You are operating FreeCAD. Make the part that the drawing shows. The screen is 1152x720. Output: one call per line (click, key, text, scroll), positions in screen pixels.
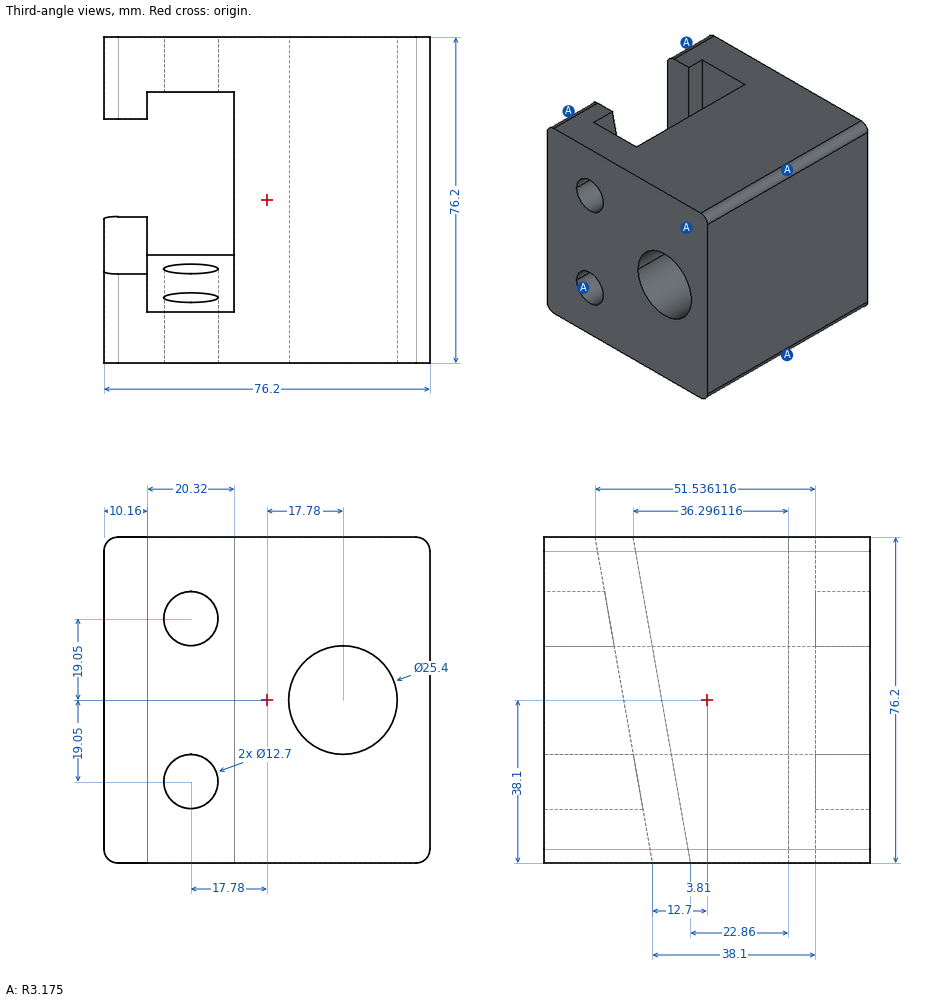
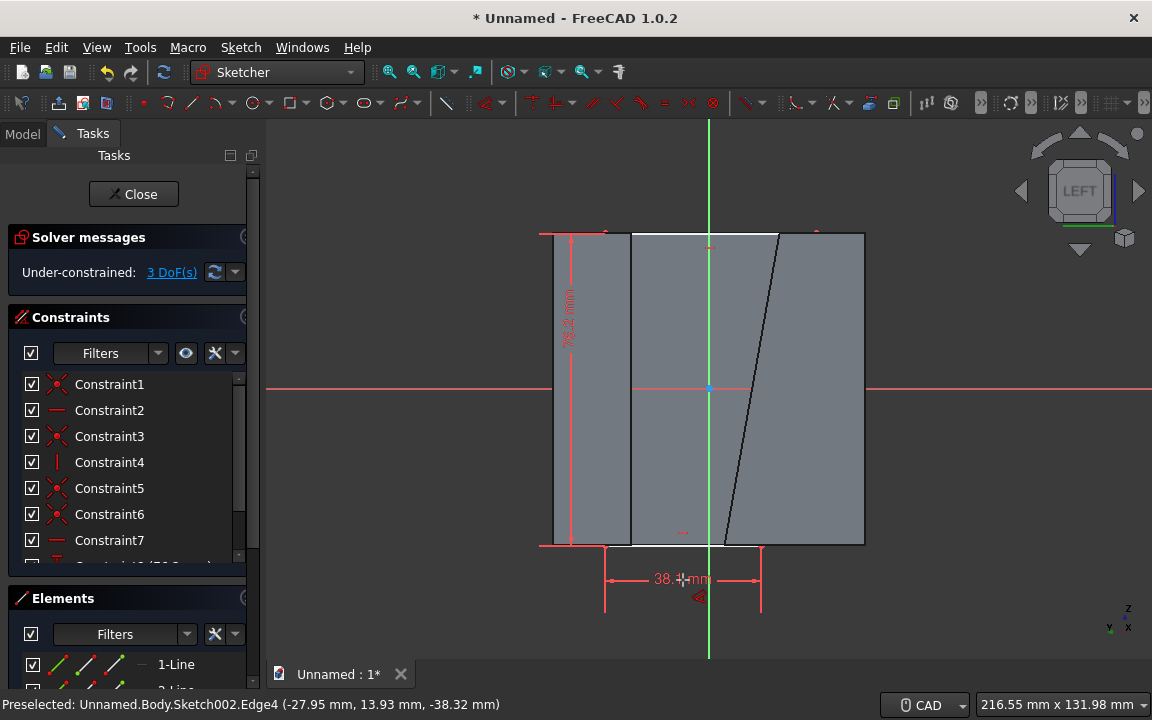
click(761, 546)
click(753, 580)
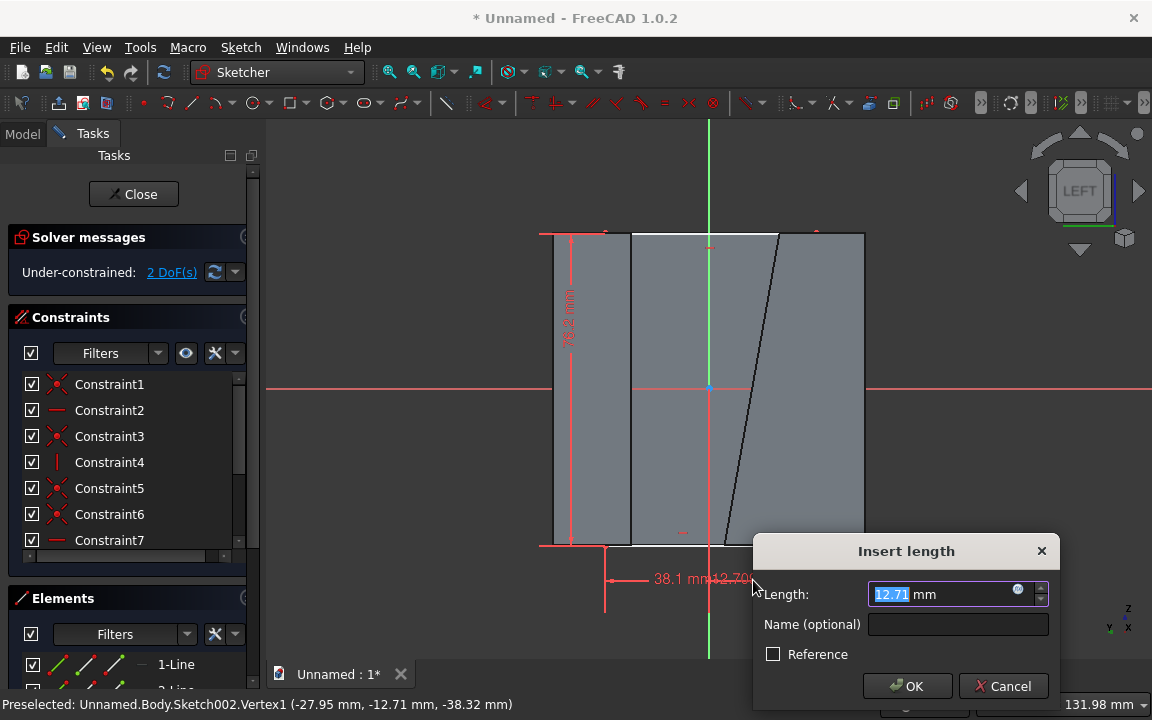
text(12.7)
key(Return)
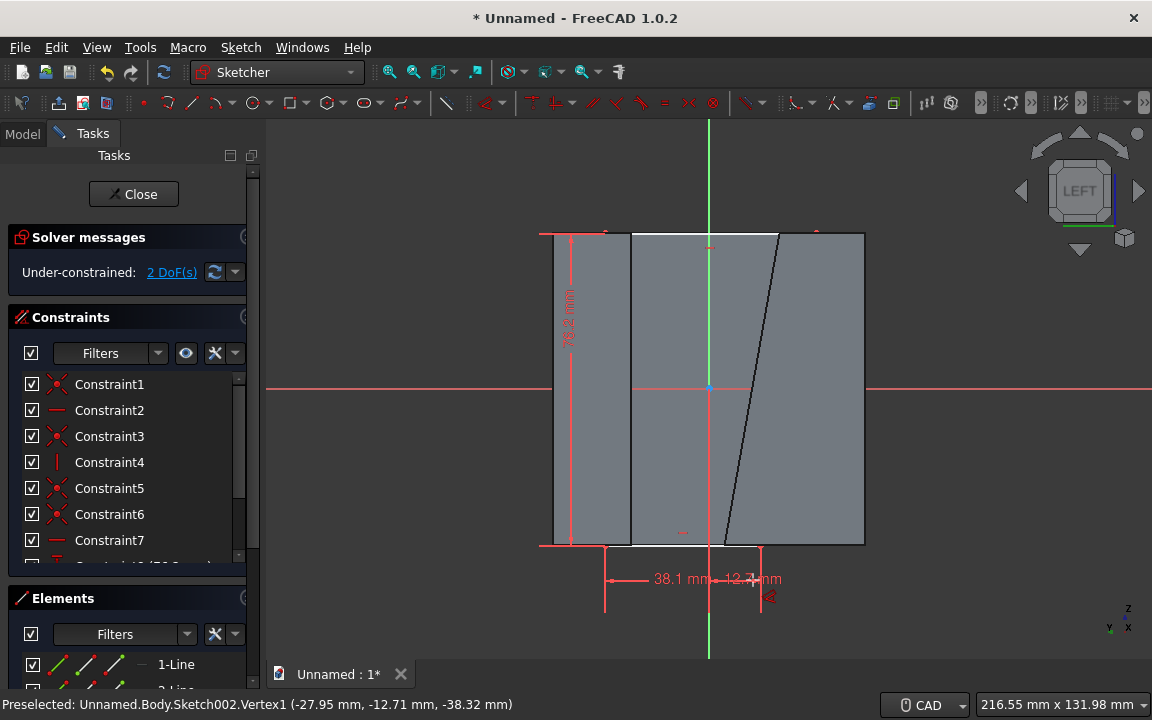
click(761, 546)
click(795, 467)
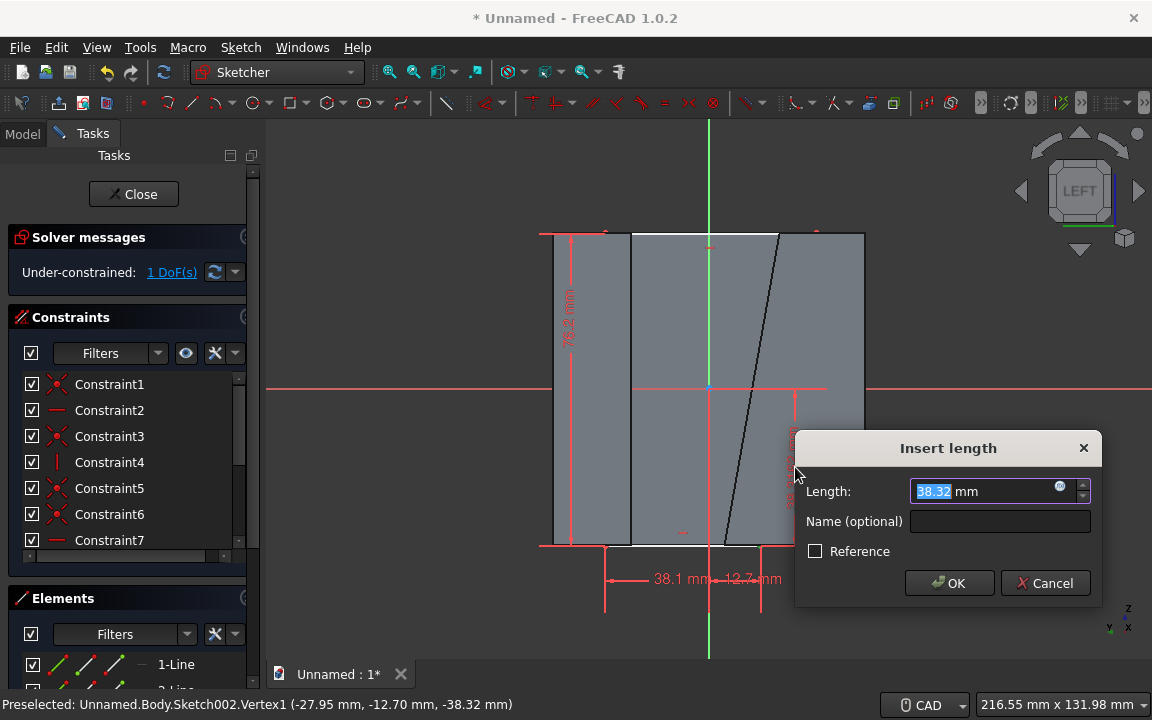
text(38.1)
key(Return)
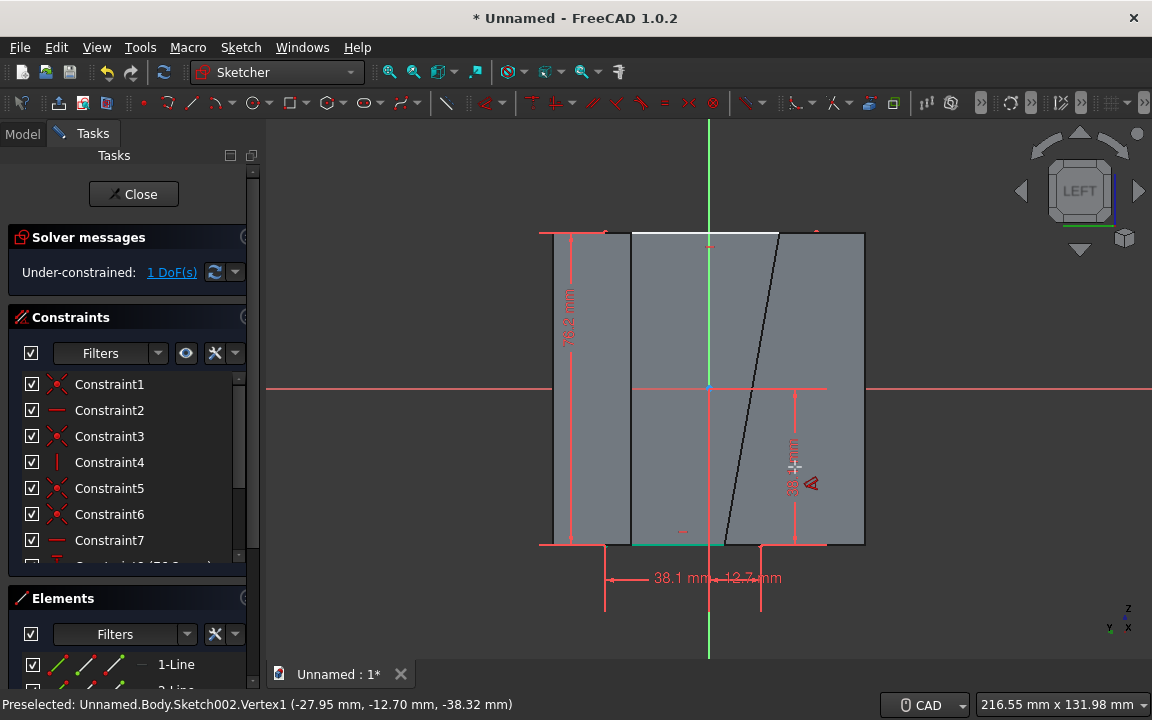
click(753, 233)
click(662, 199)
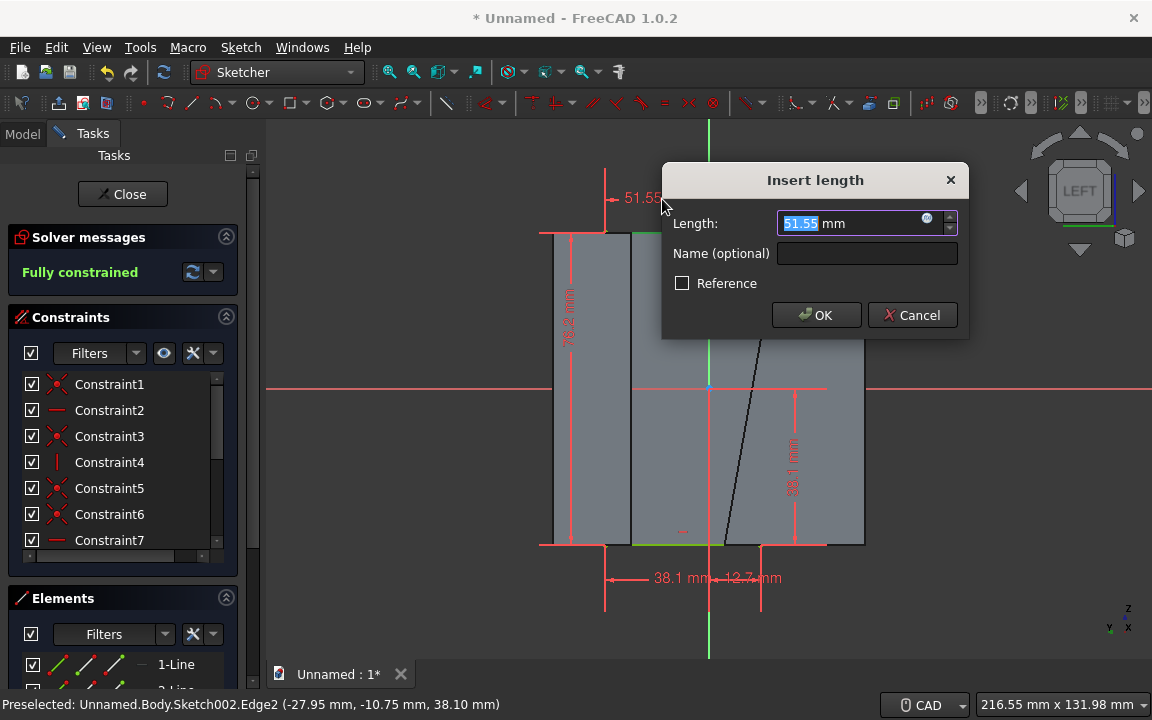
text(51.536116)
key(Return)
key(Escape)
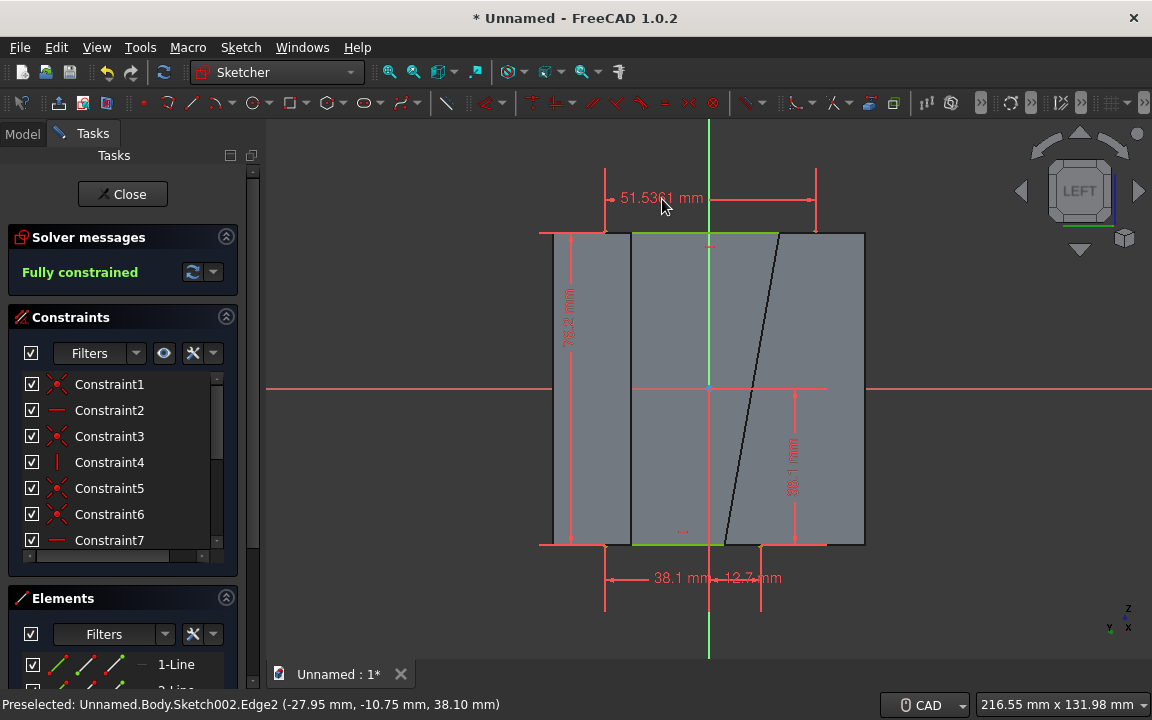
click(123, 194)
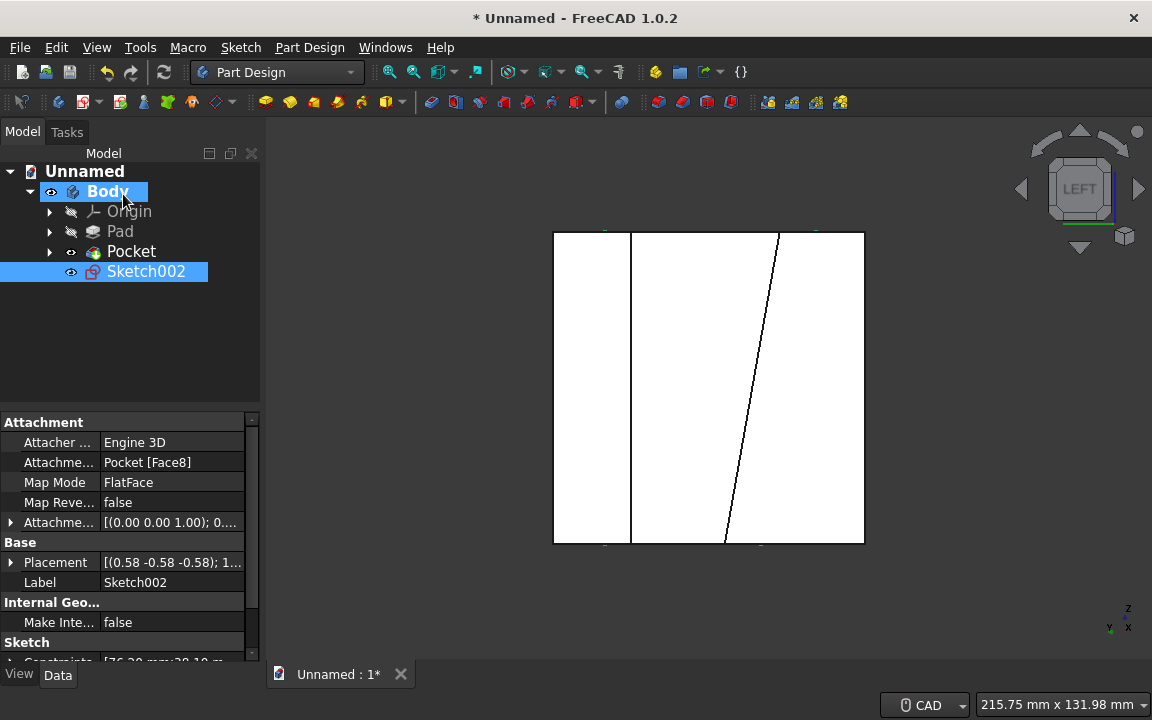
click(432, 102)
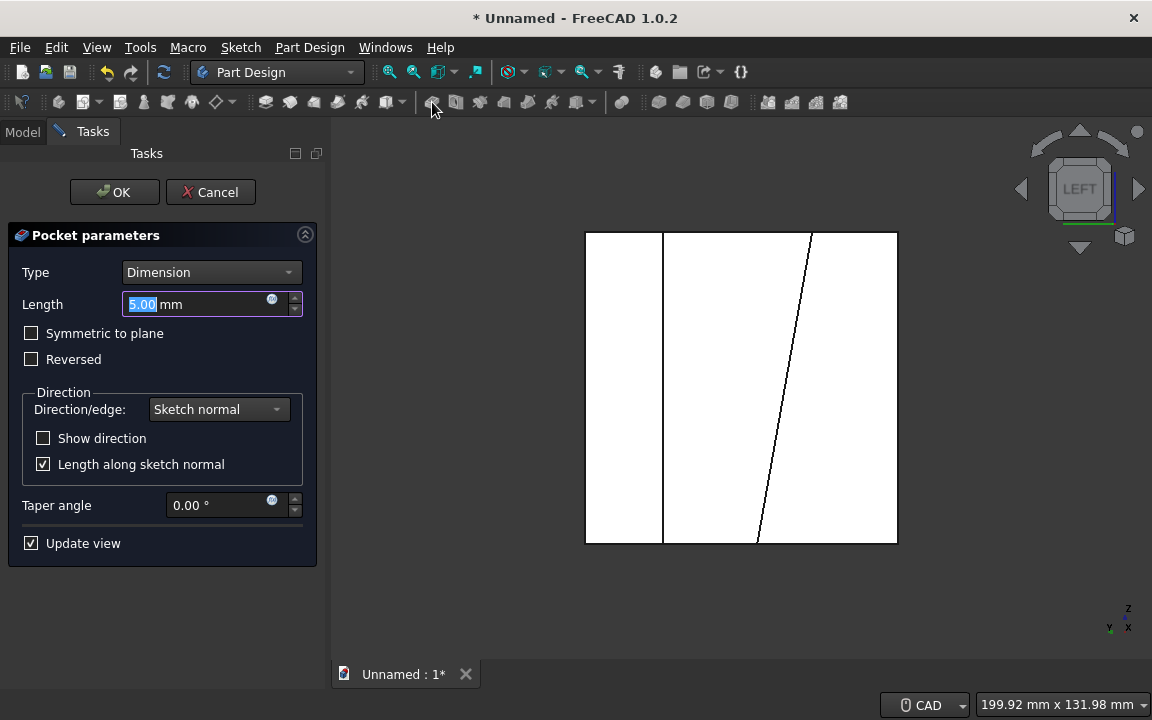
text(20.32)
key(Tab)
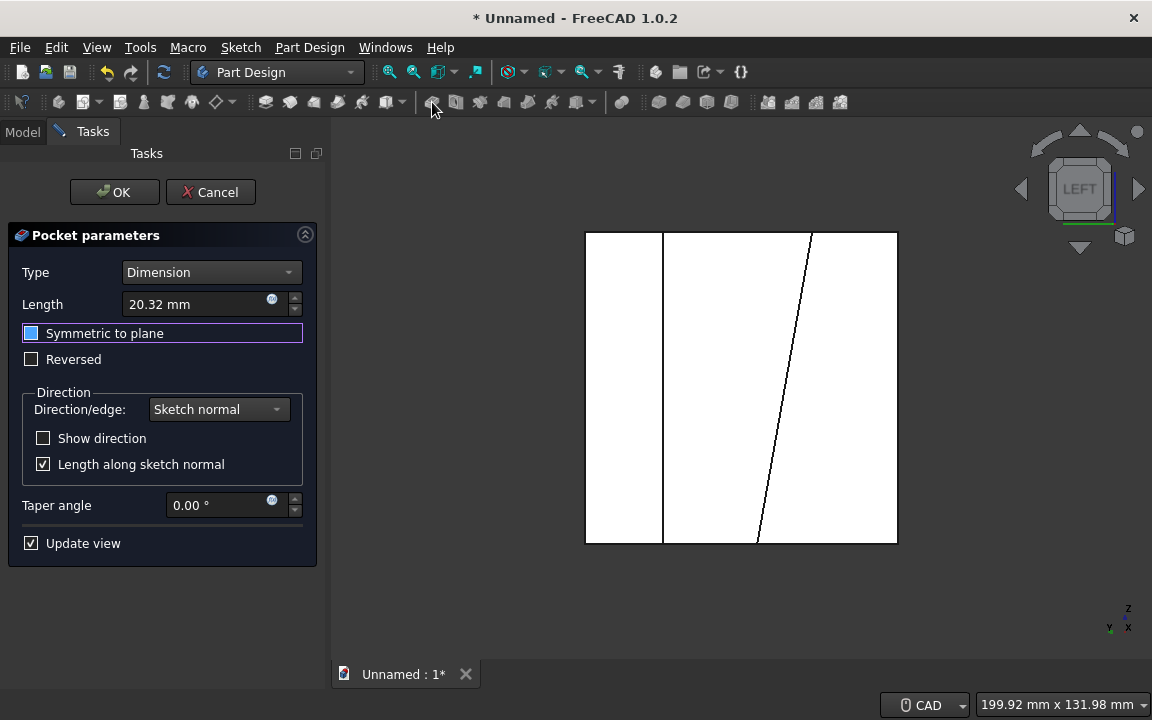
click(115, 192)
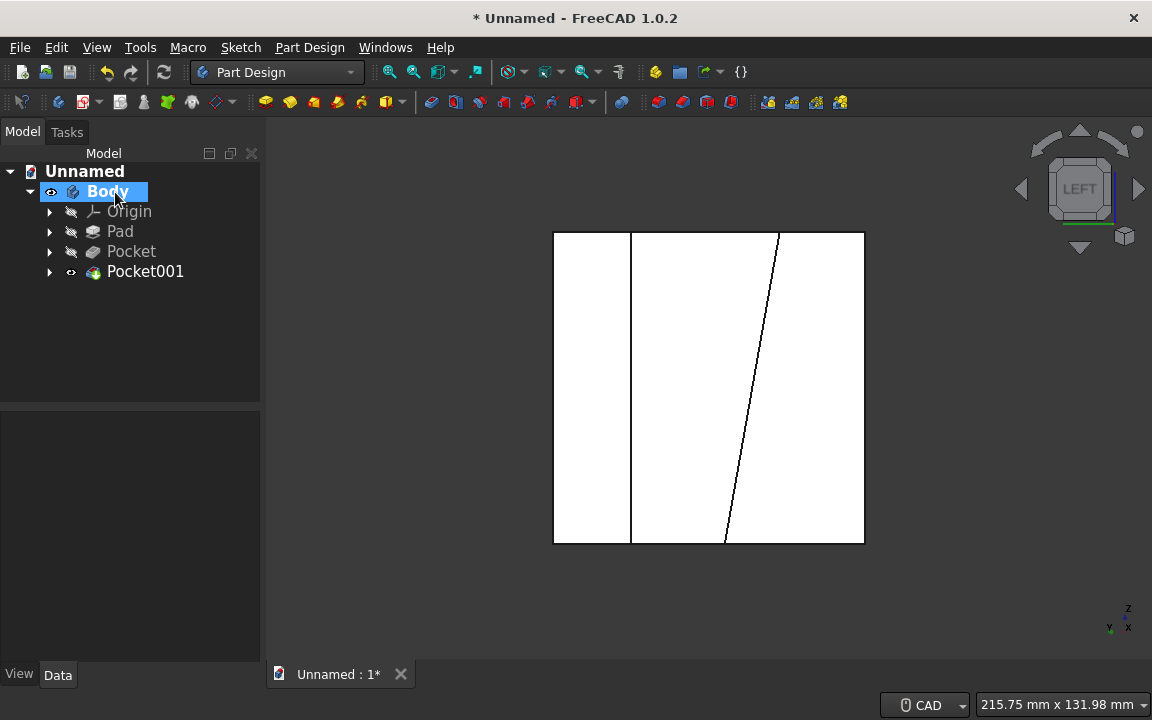
click(592, 231)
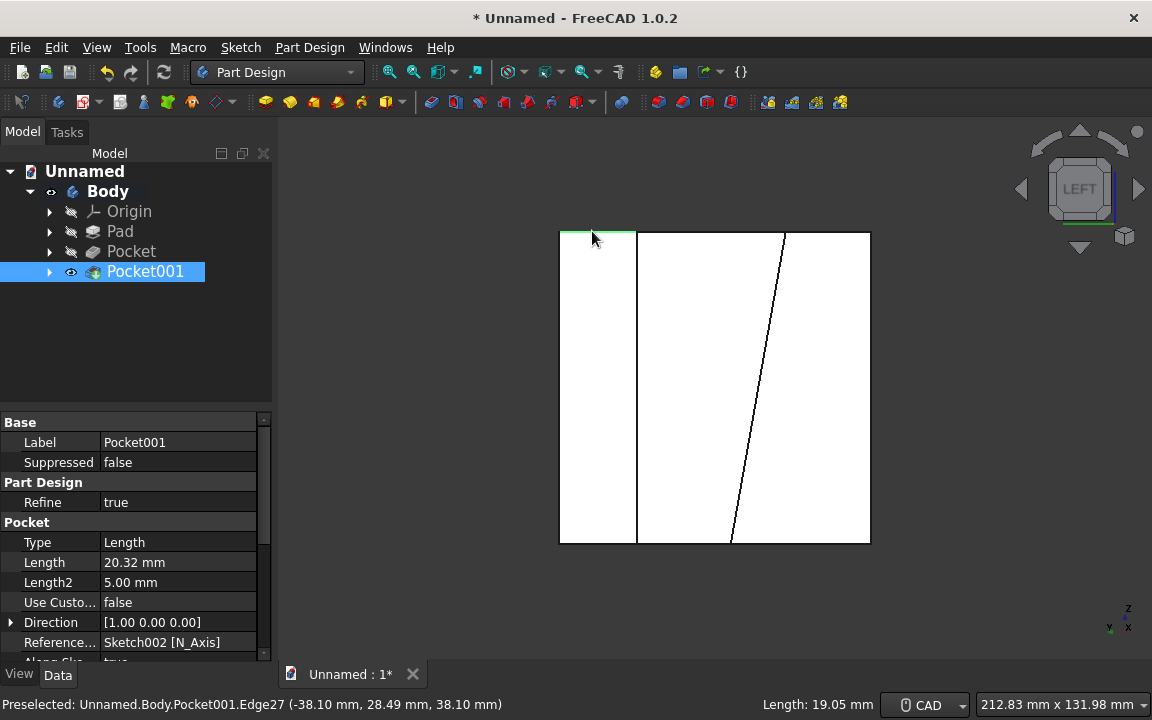
click(801, 543, ctrl)